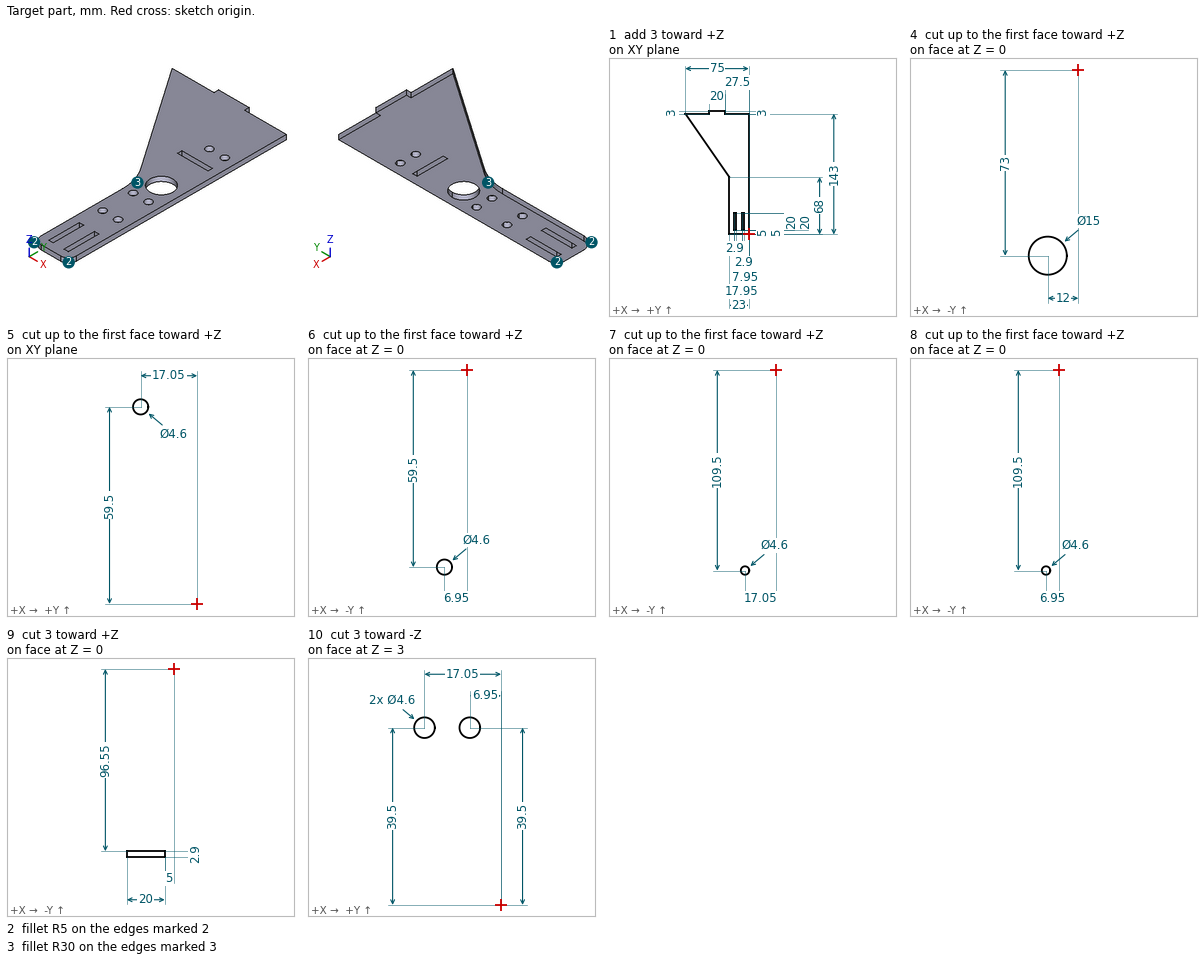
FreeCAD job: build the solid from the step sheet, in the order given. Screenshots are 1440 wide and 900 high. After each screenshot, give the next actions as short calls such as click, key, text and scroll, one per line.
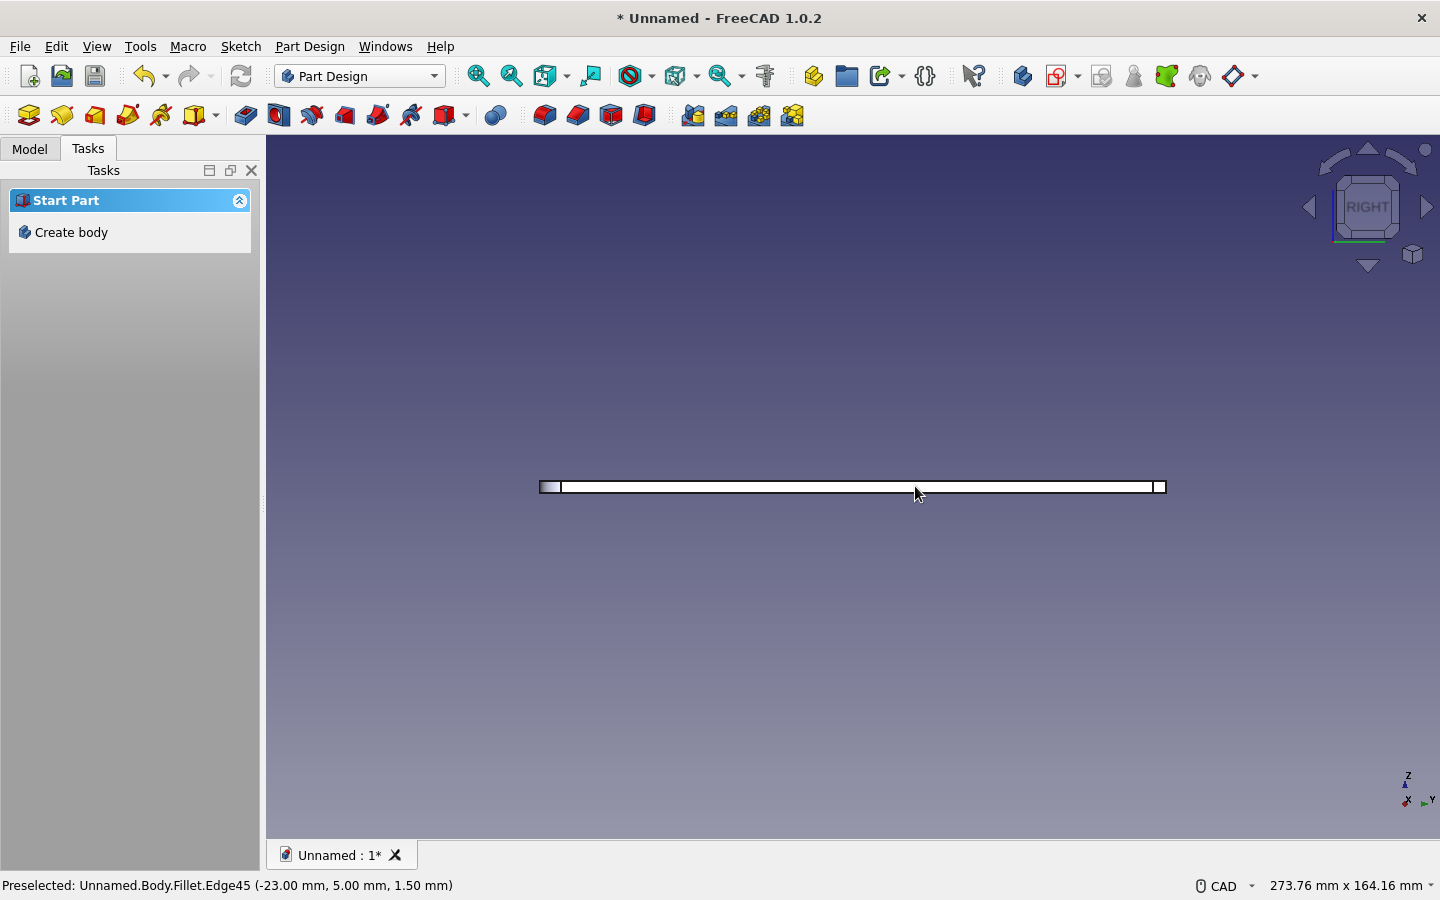
scroll(832, 486, up, 6)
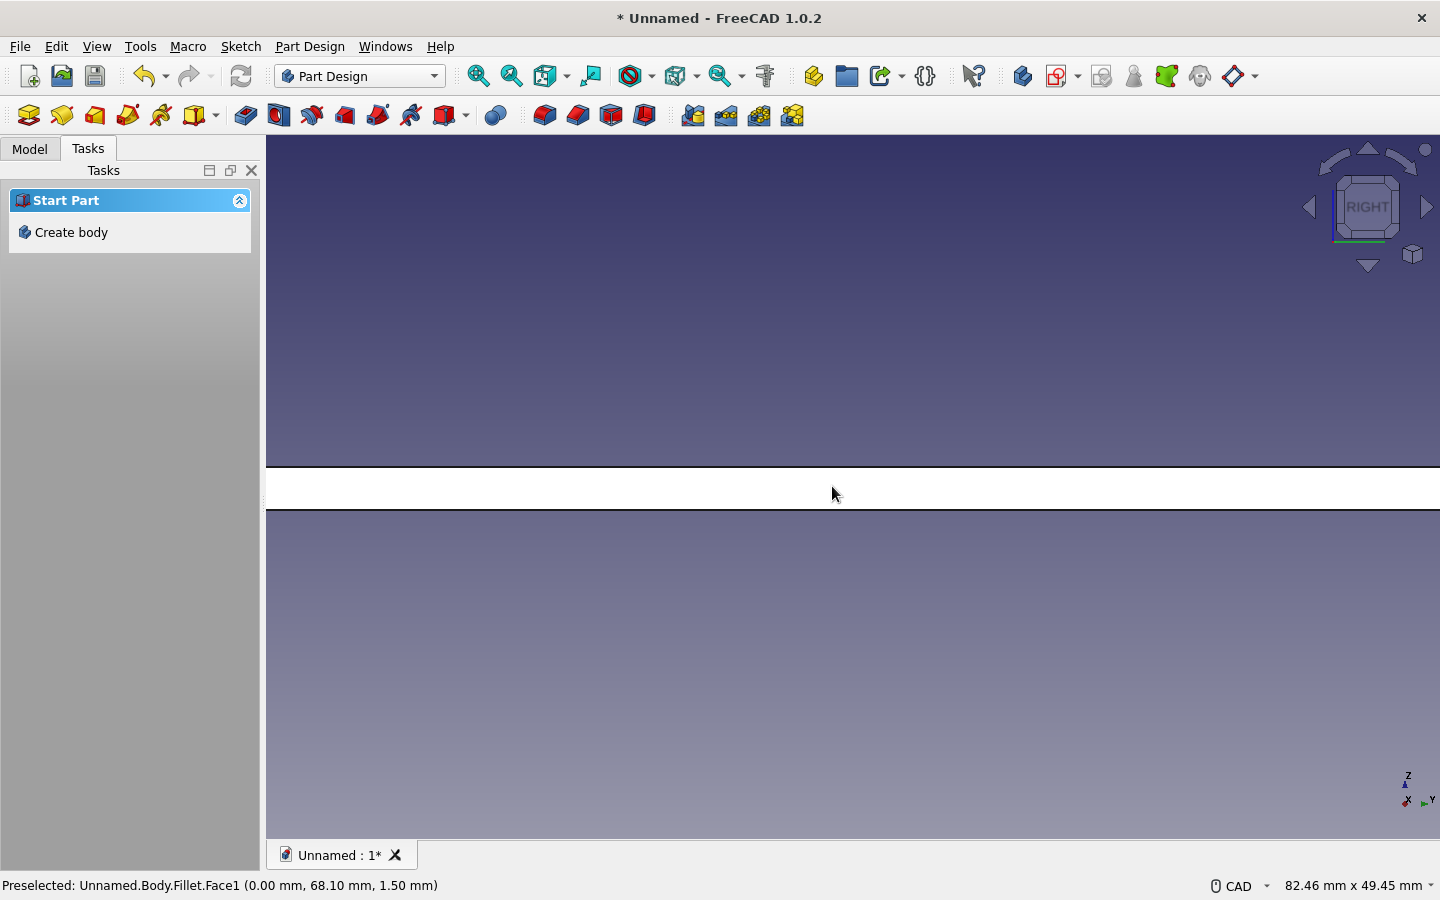
key(v)
key(f)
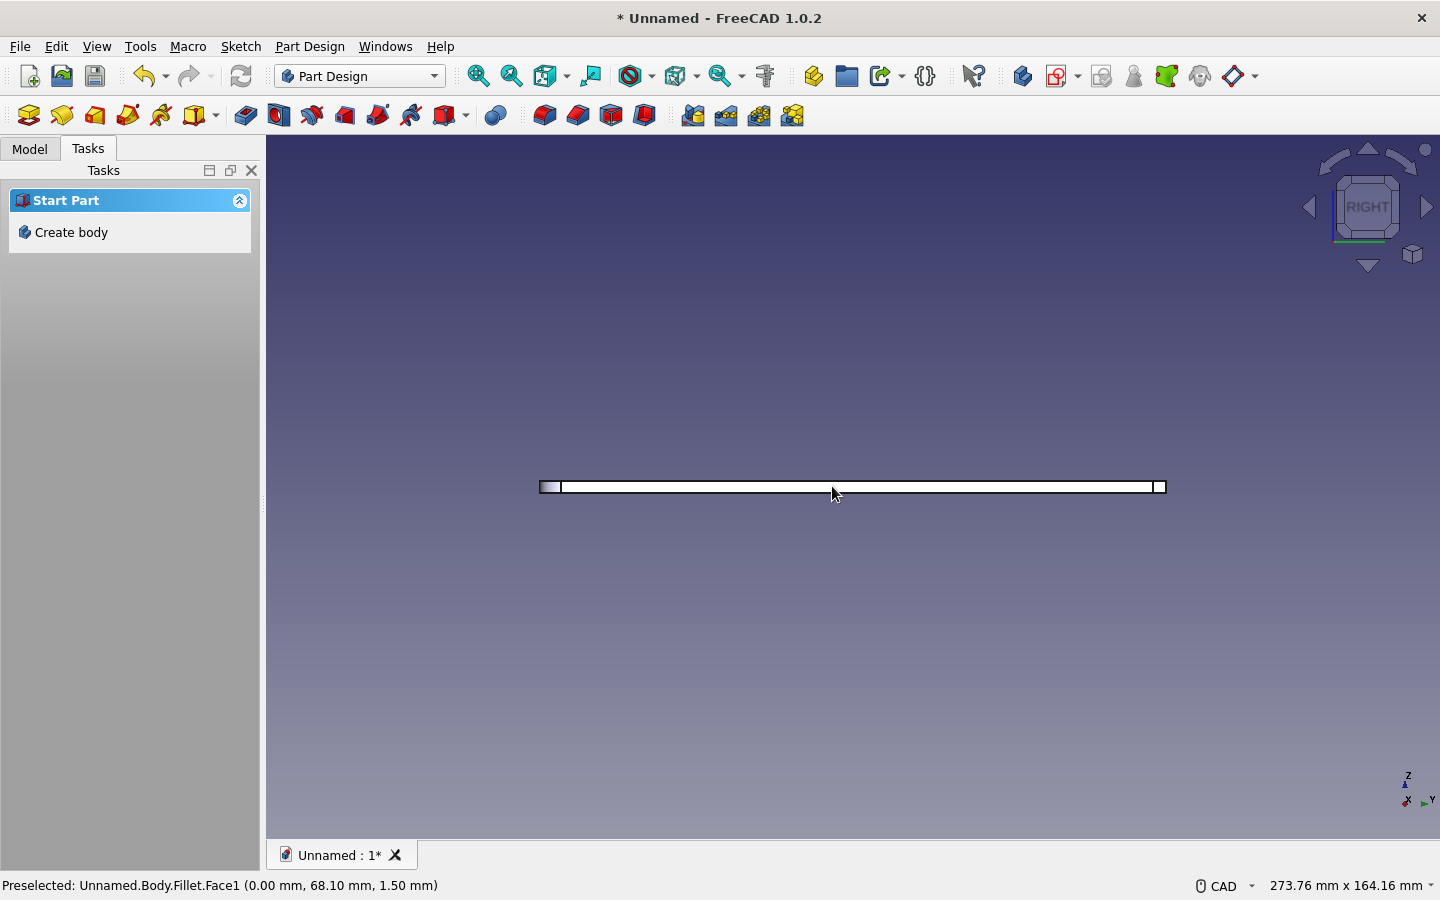
key(5)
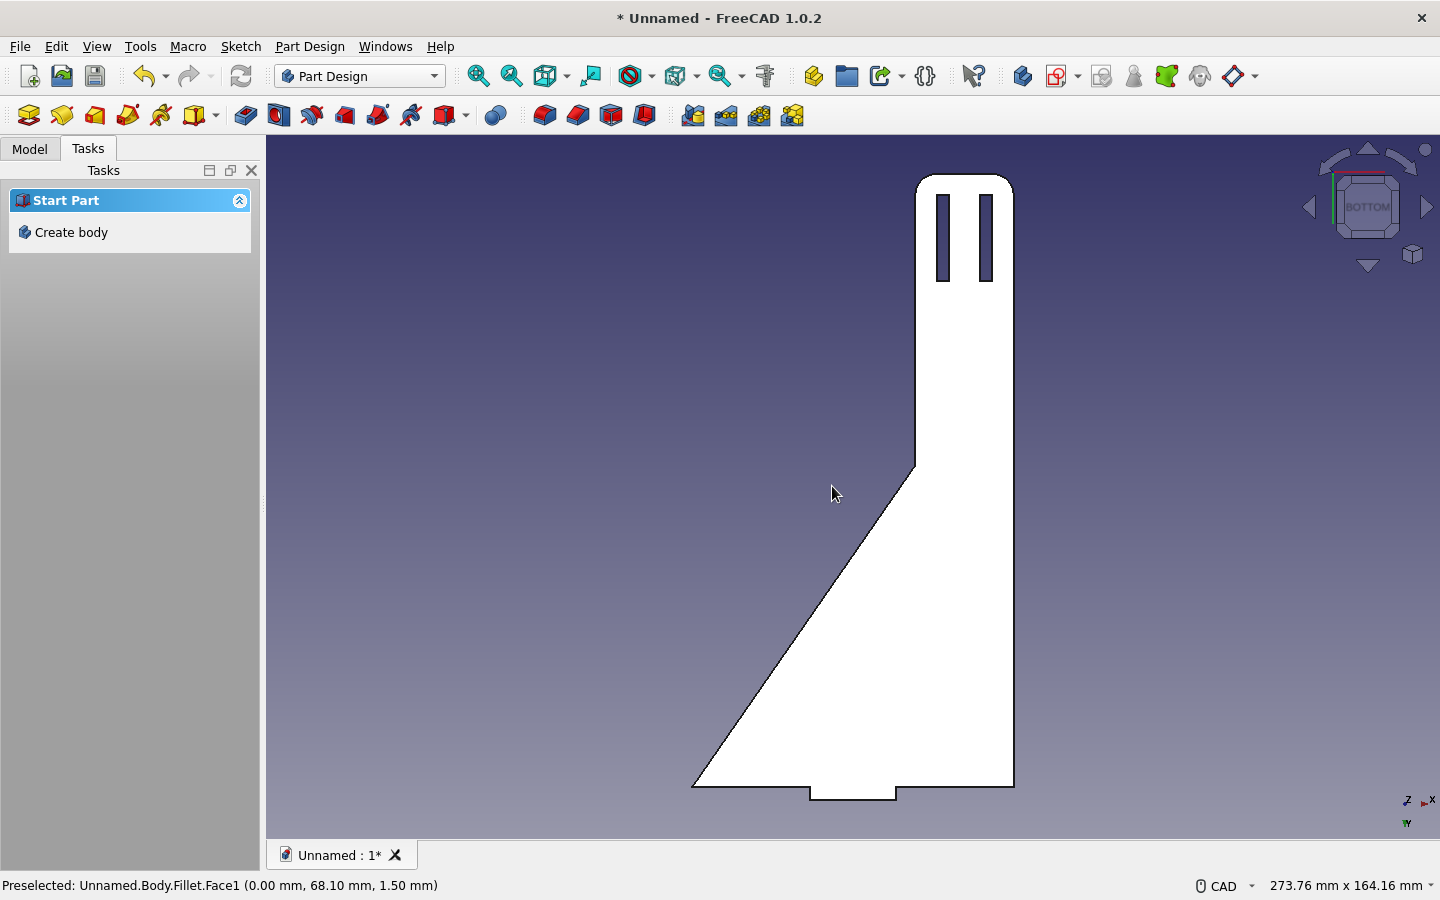
scroll(915, 465, up, 6)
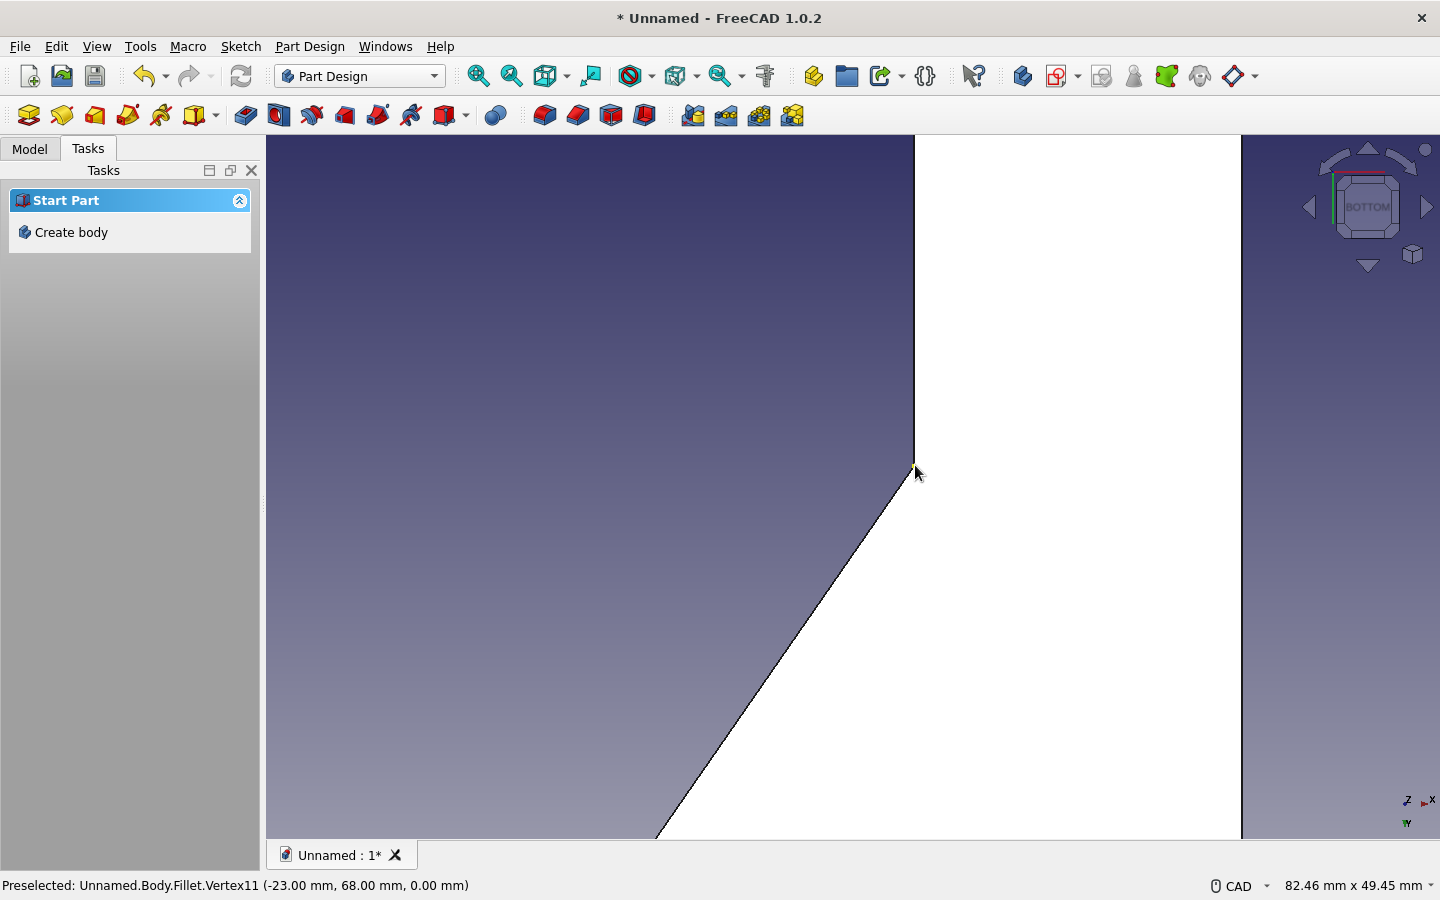
key(v)
key(f)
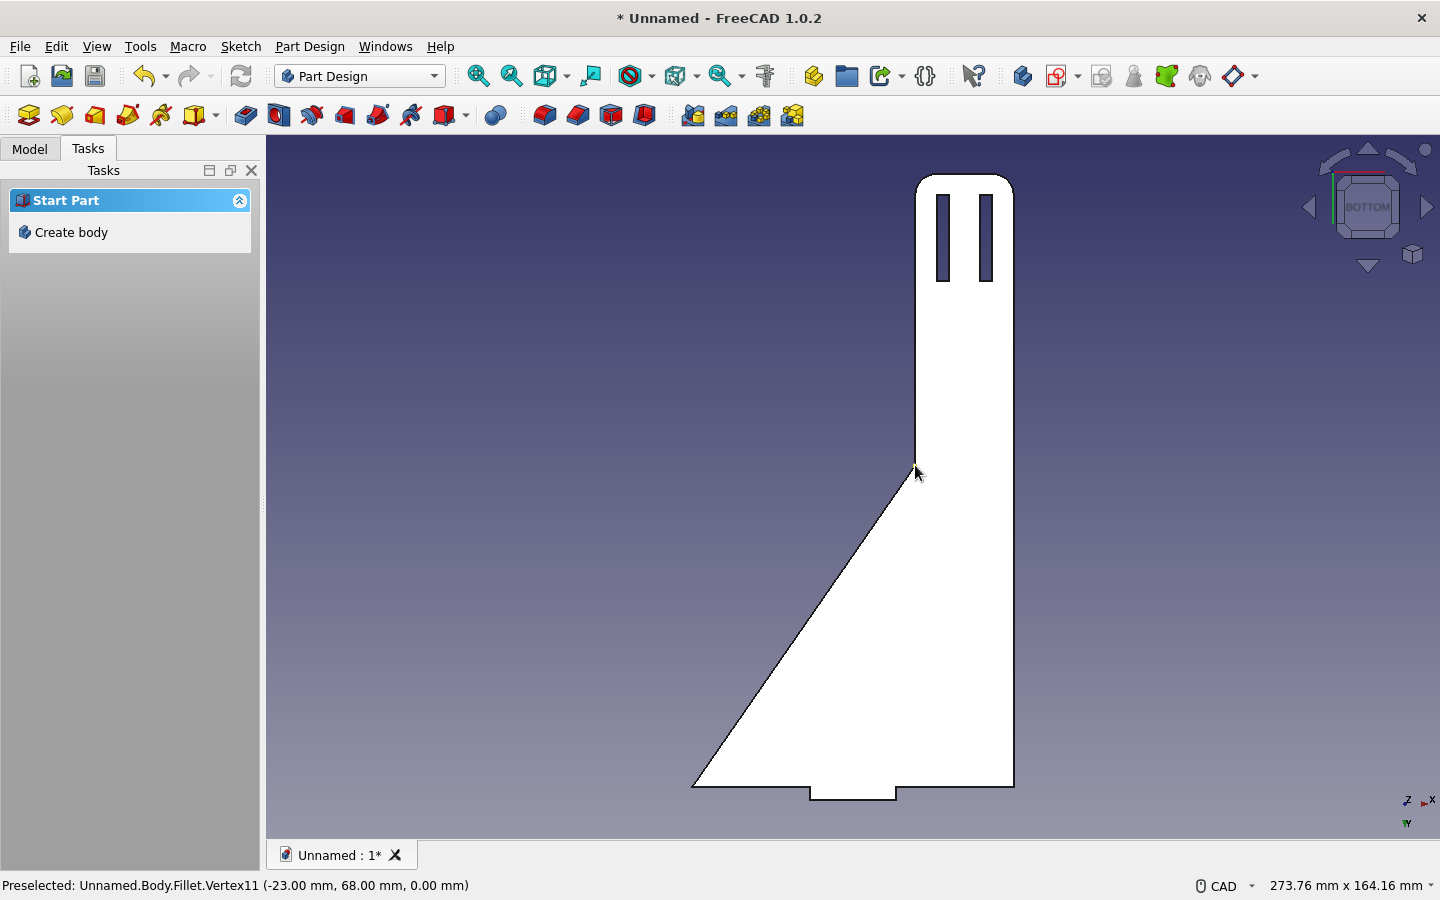
key(4)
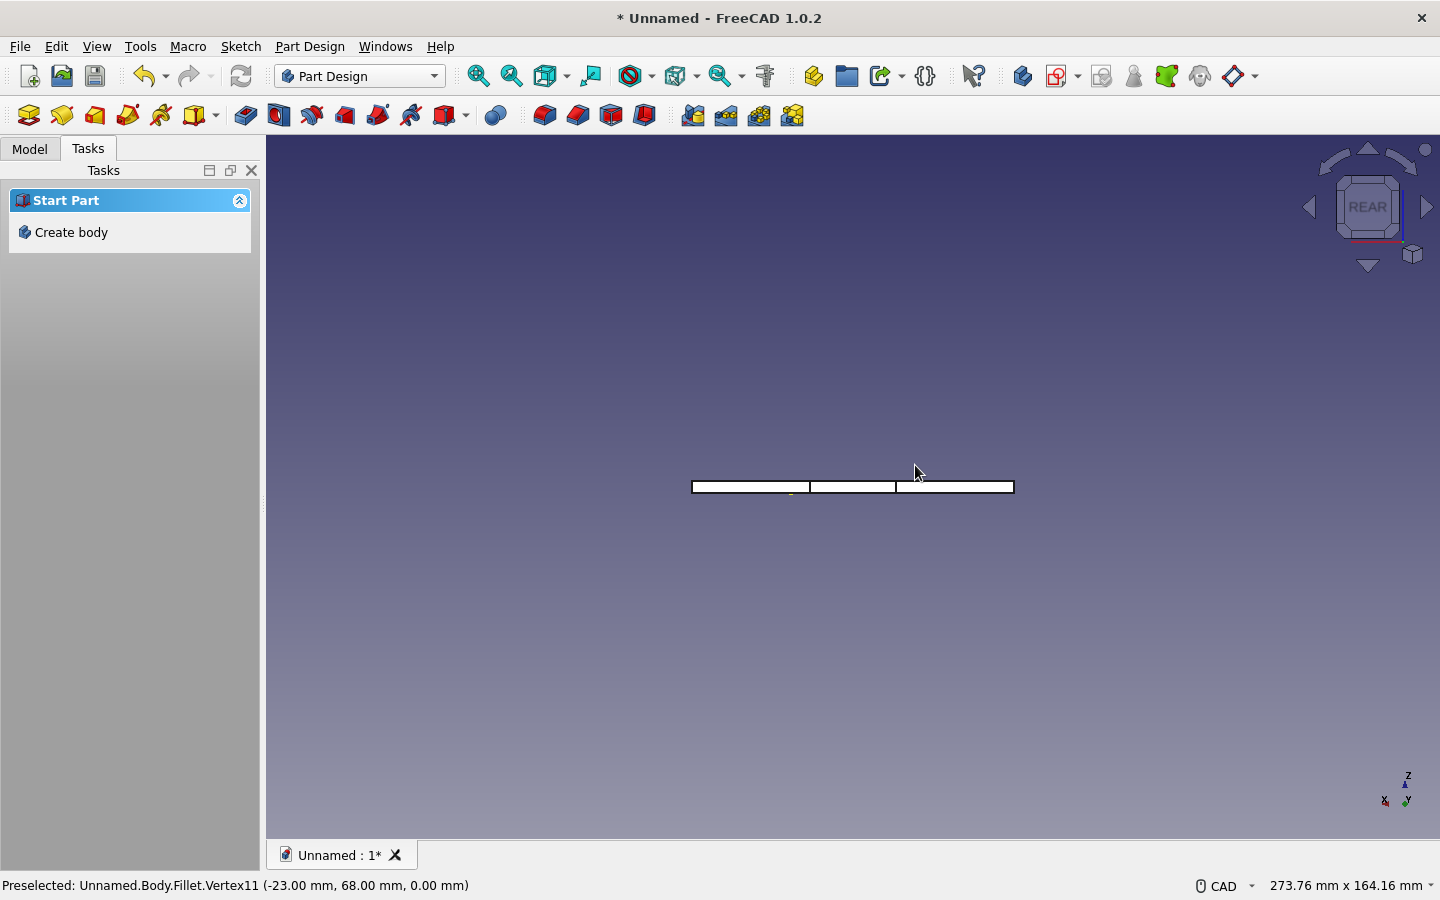
key(v)
key(f)